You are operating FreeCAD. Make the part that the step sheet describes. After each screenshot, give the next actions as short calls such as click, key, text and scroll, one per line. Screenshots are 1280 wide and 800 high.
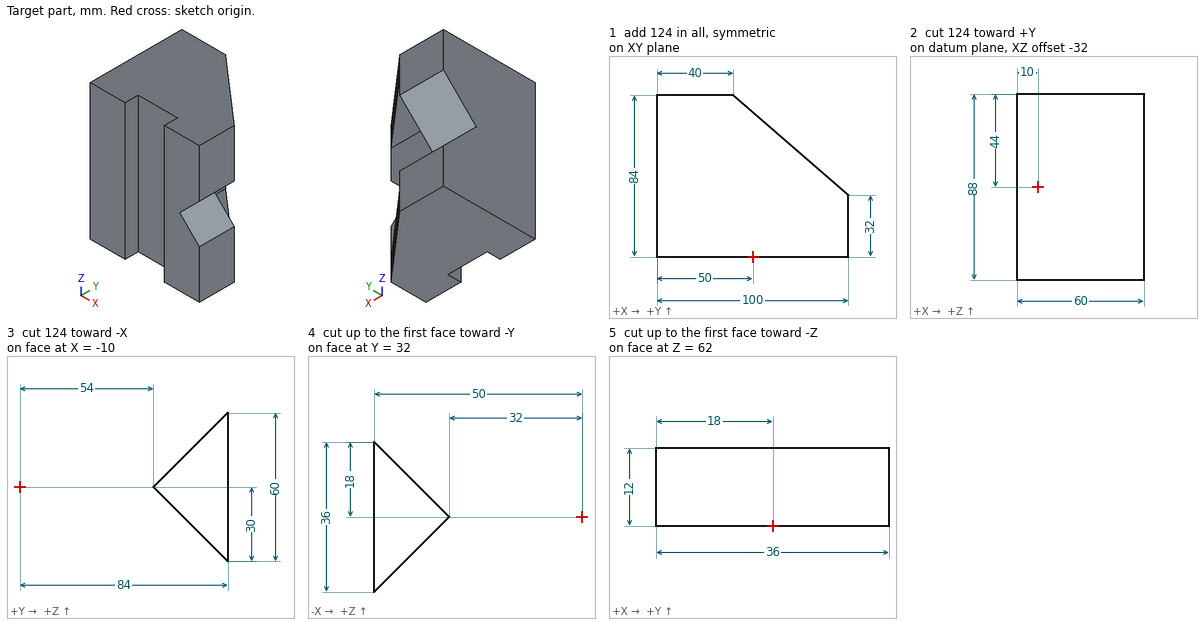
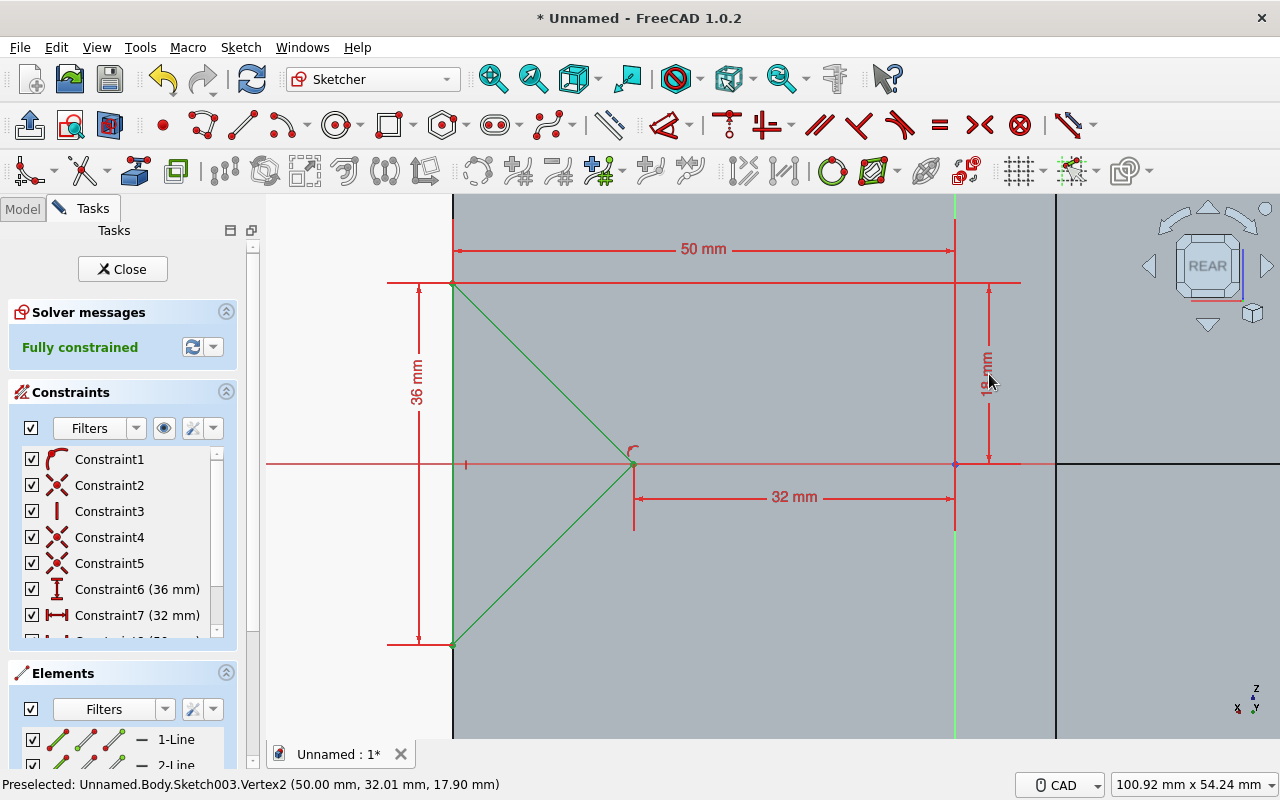
click(123, 269)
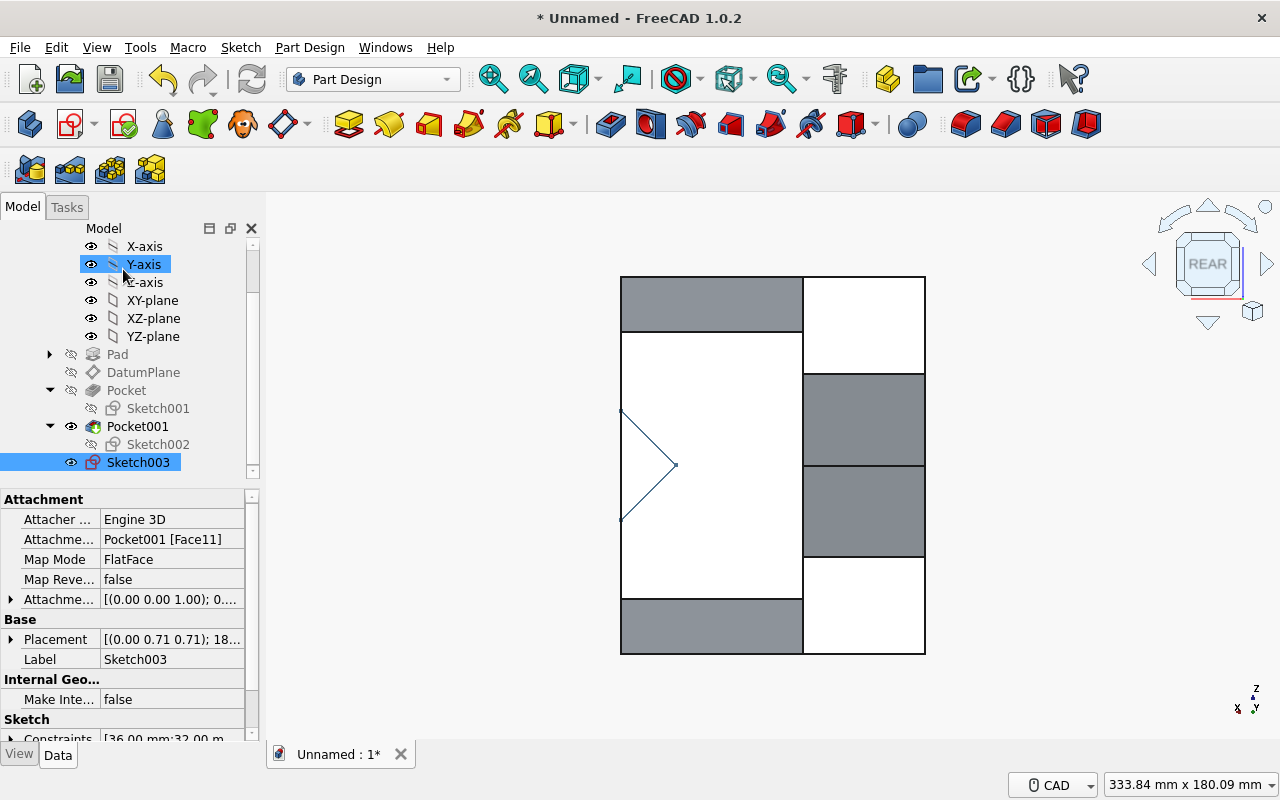
click(612, 124)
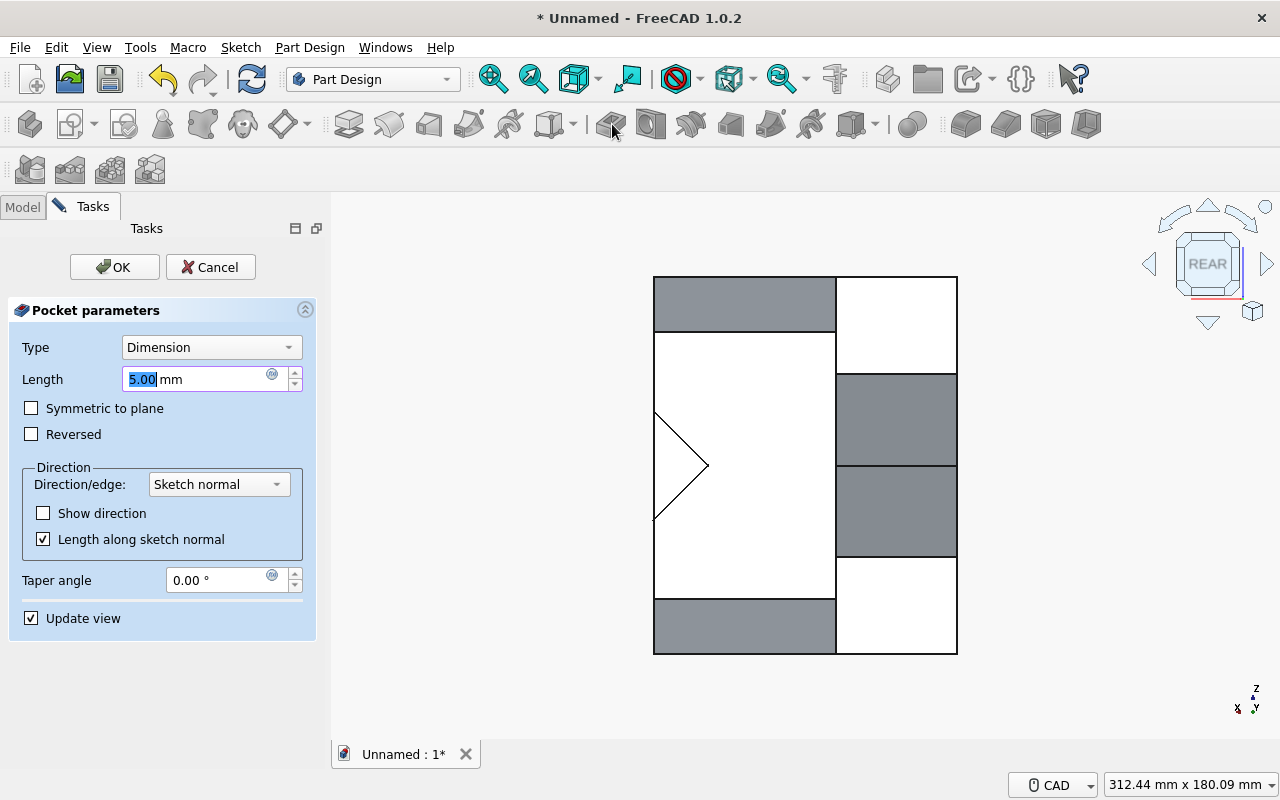
click(212, 348)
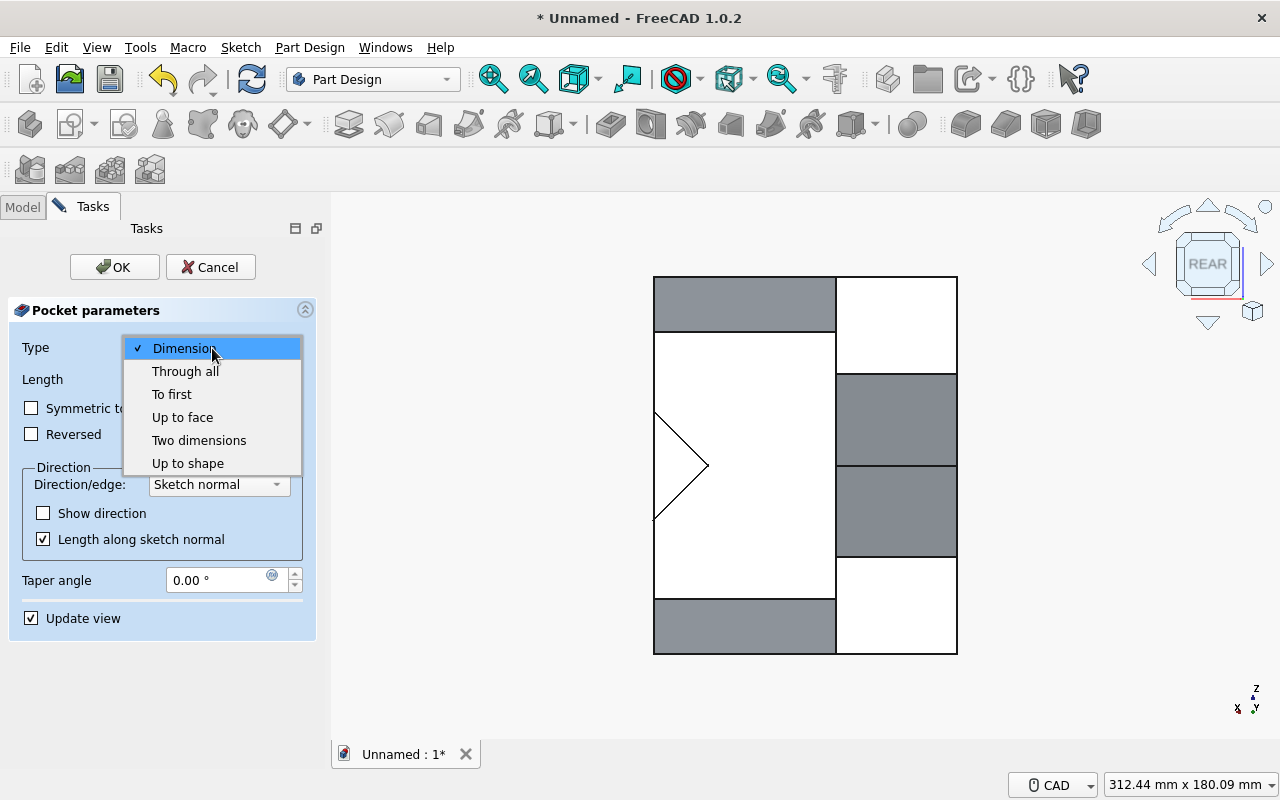
click(212, 394)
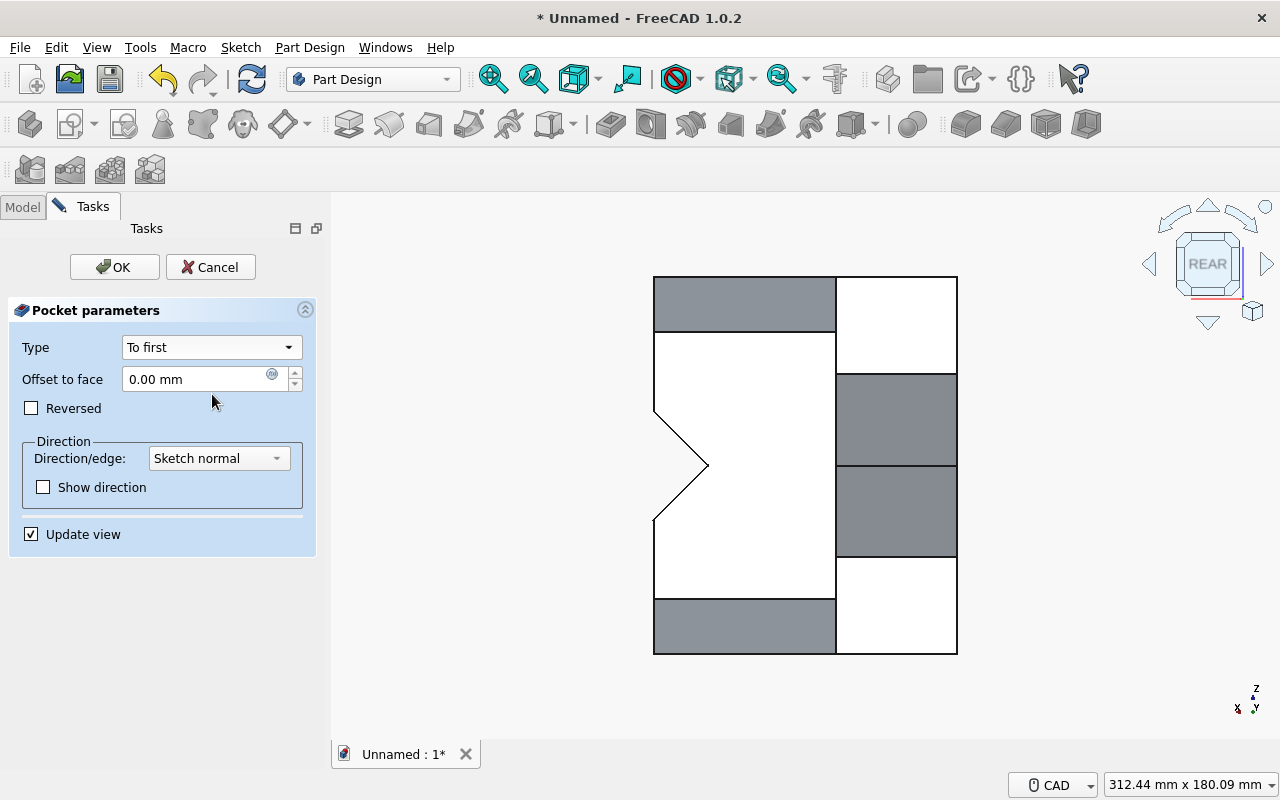
click(115, 267)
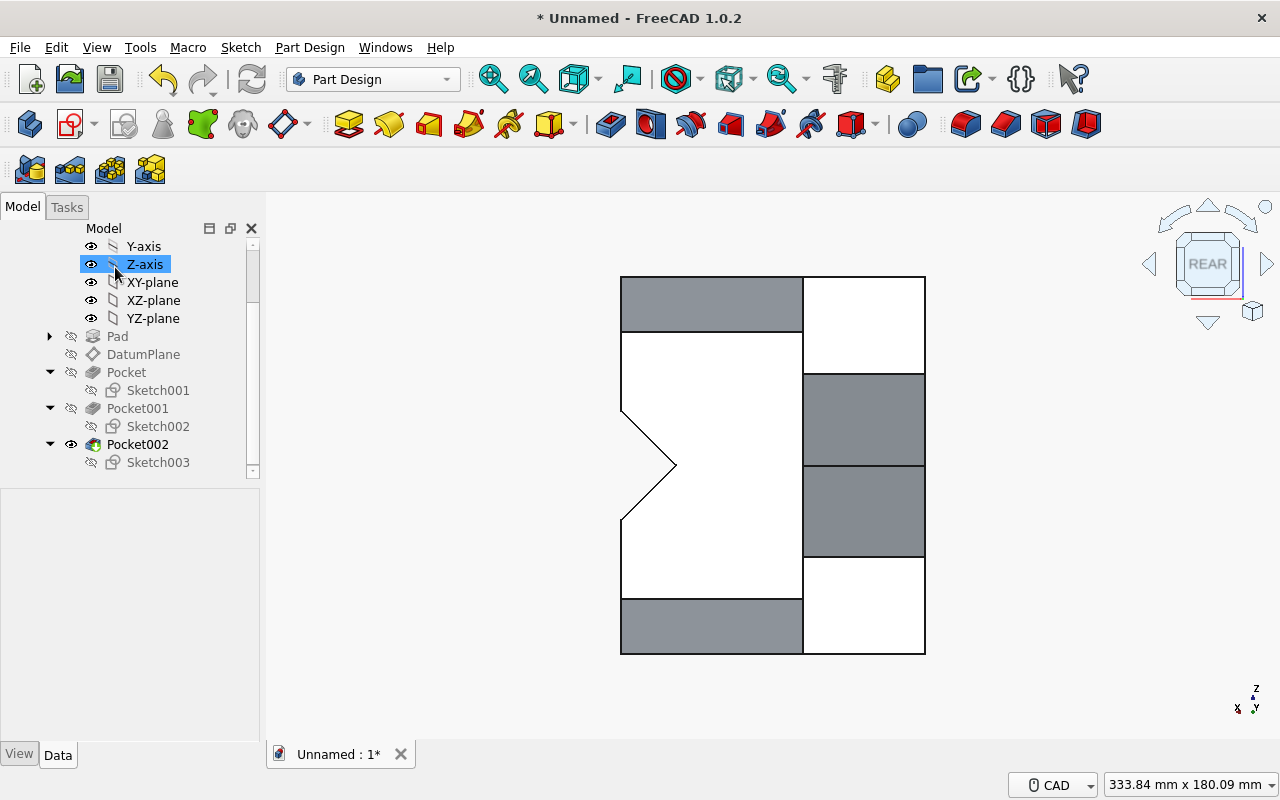
key(0)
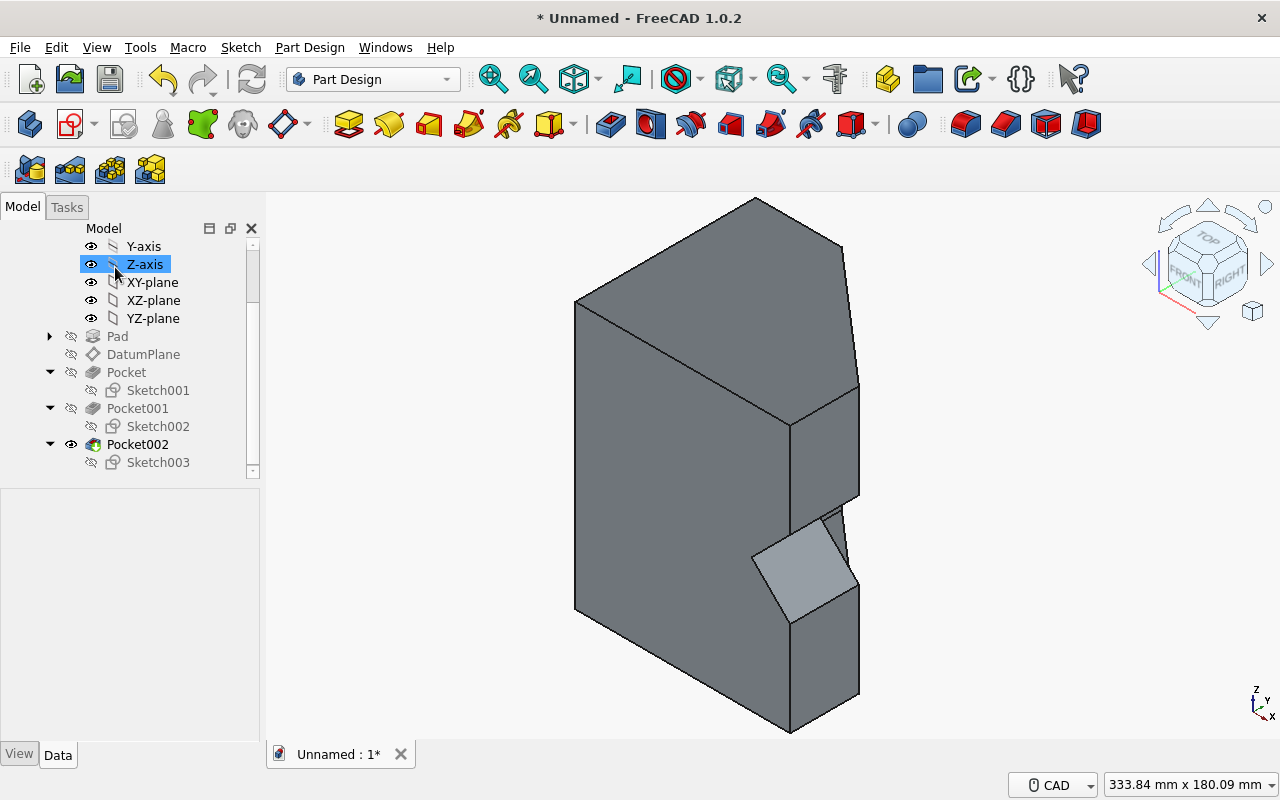
click(742, 293)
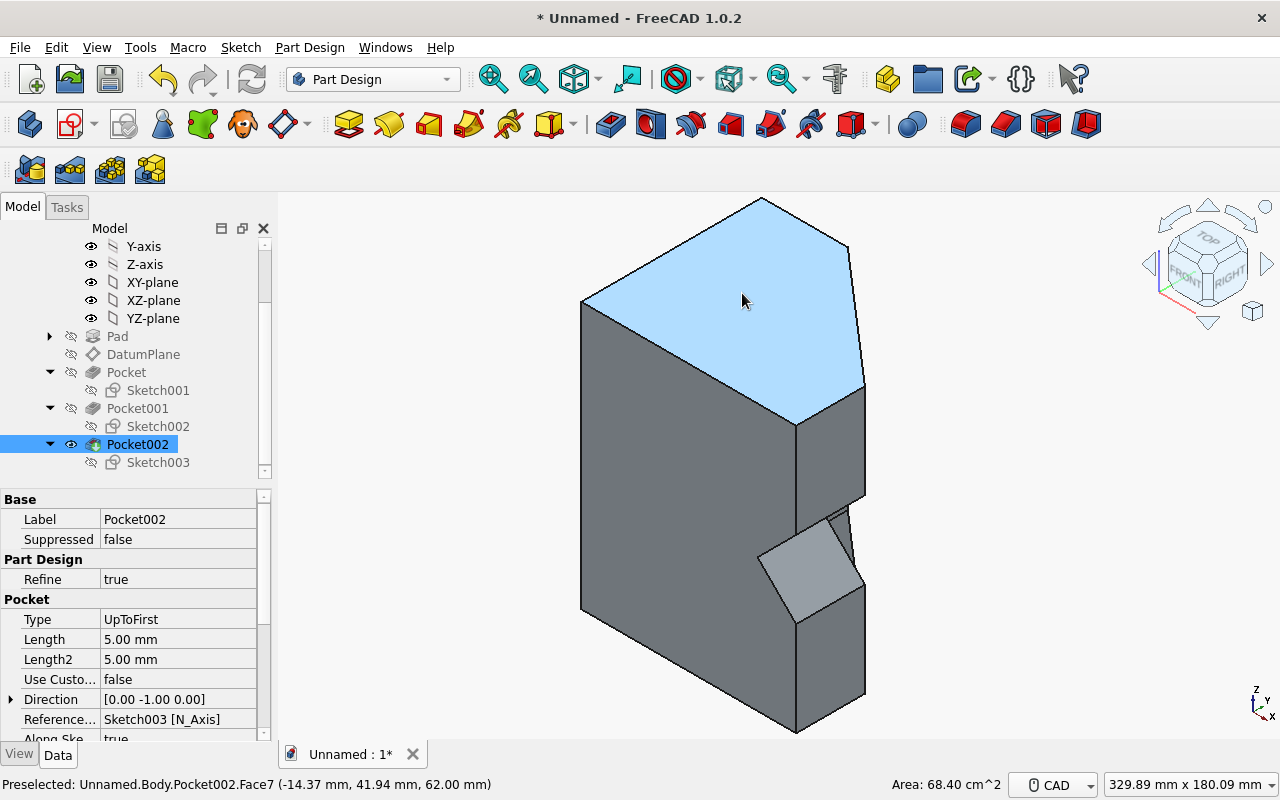
click(70, 124)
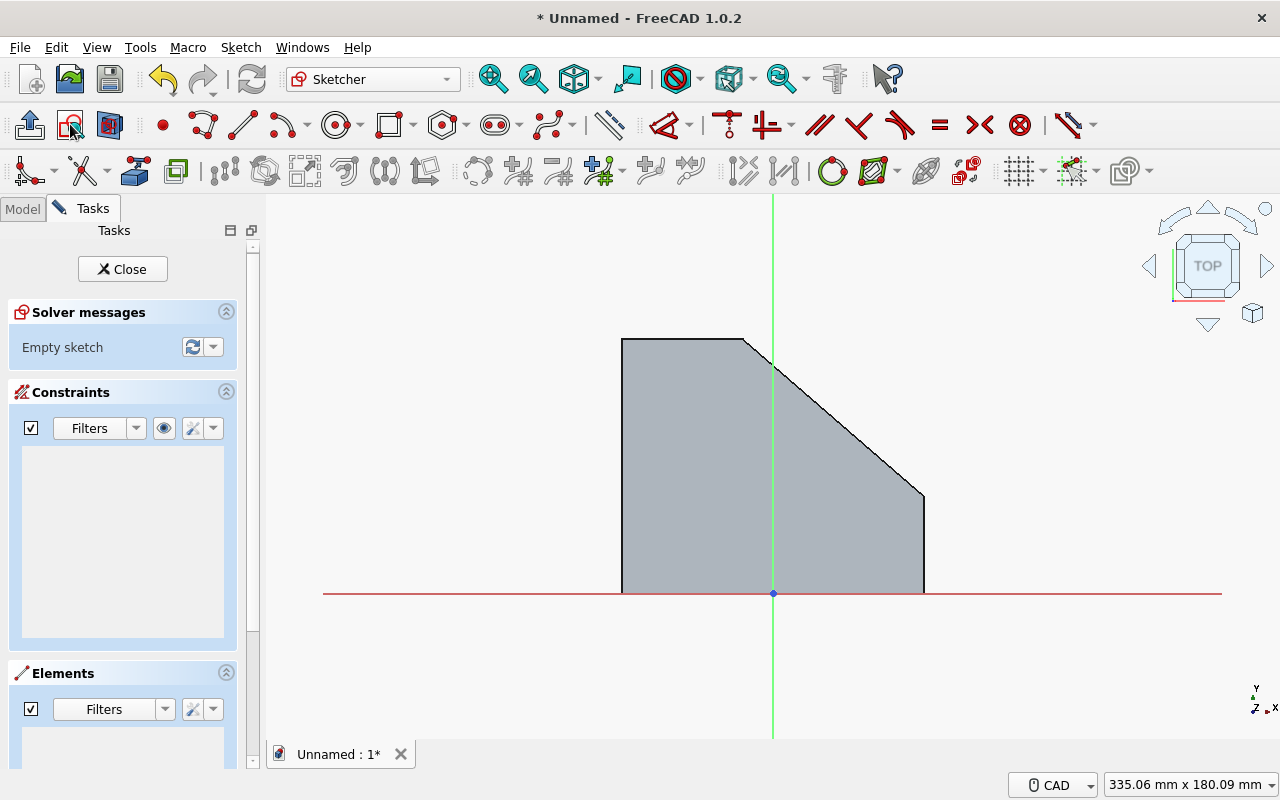
scroll(790, 603, up, 8)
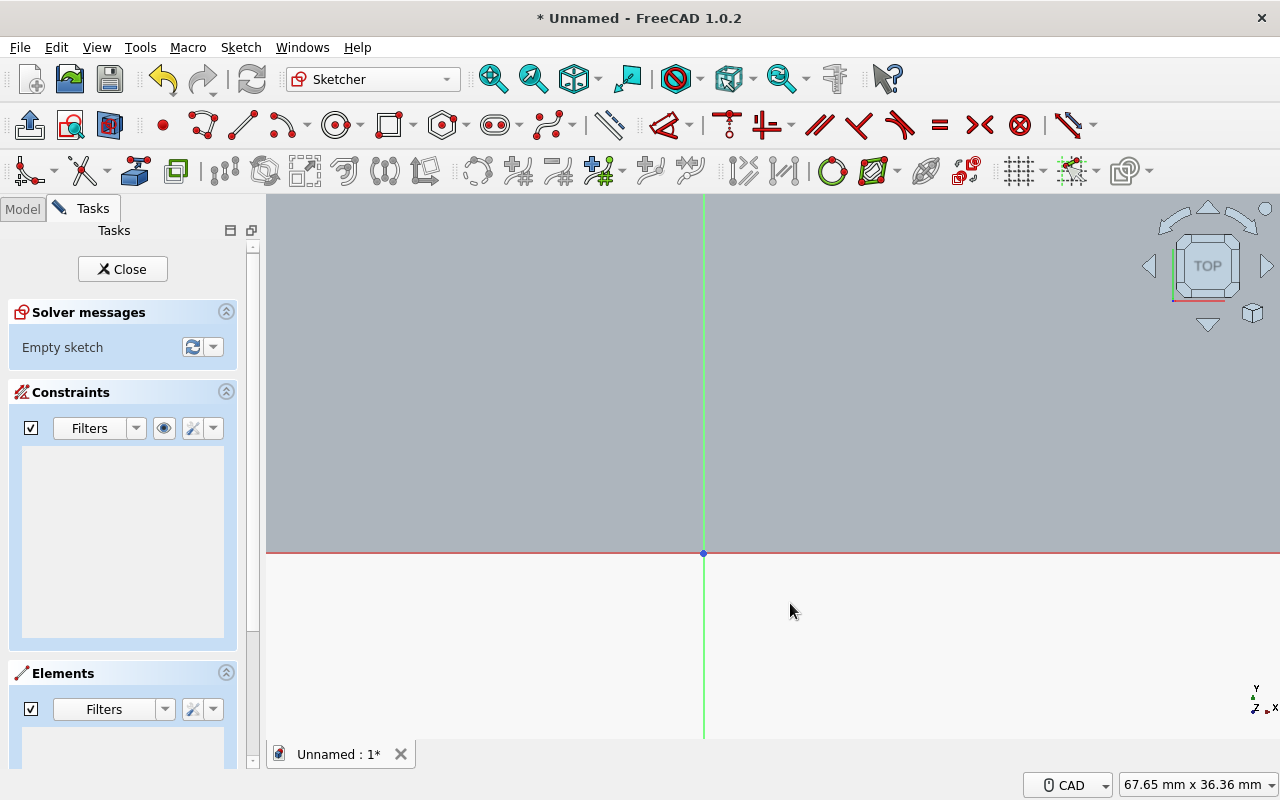
click(390, 126)